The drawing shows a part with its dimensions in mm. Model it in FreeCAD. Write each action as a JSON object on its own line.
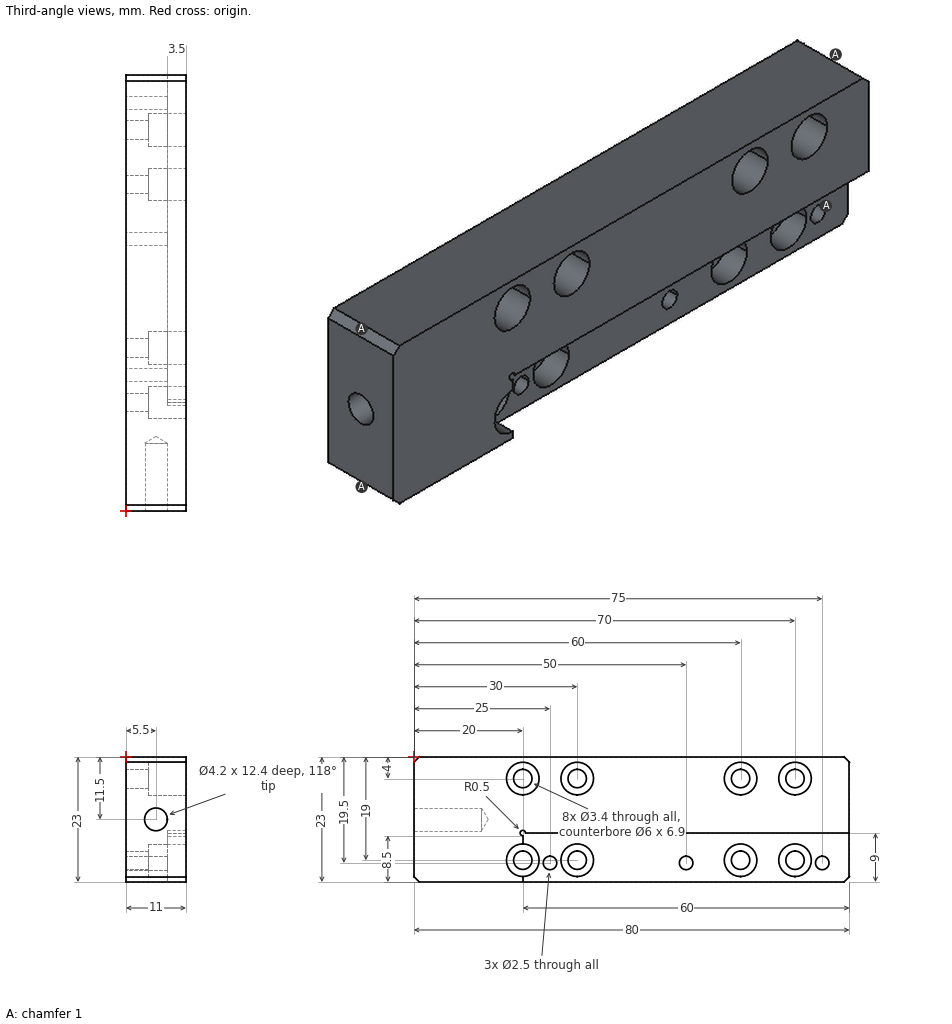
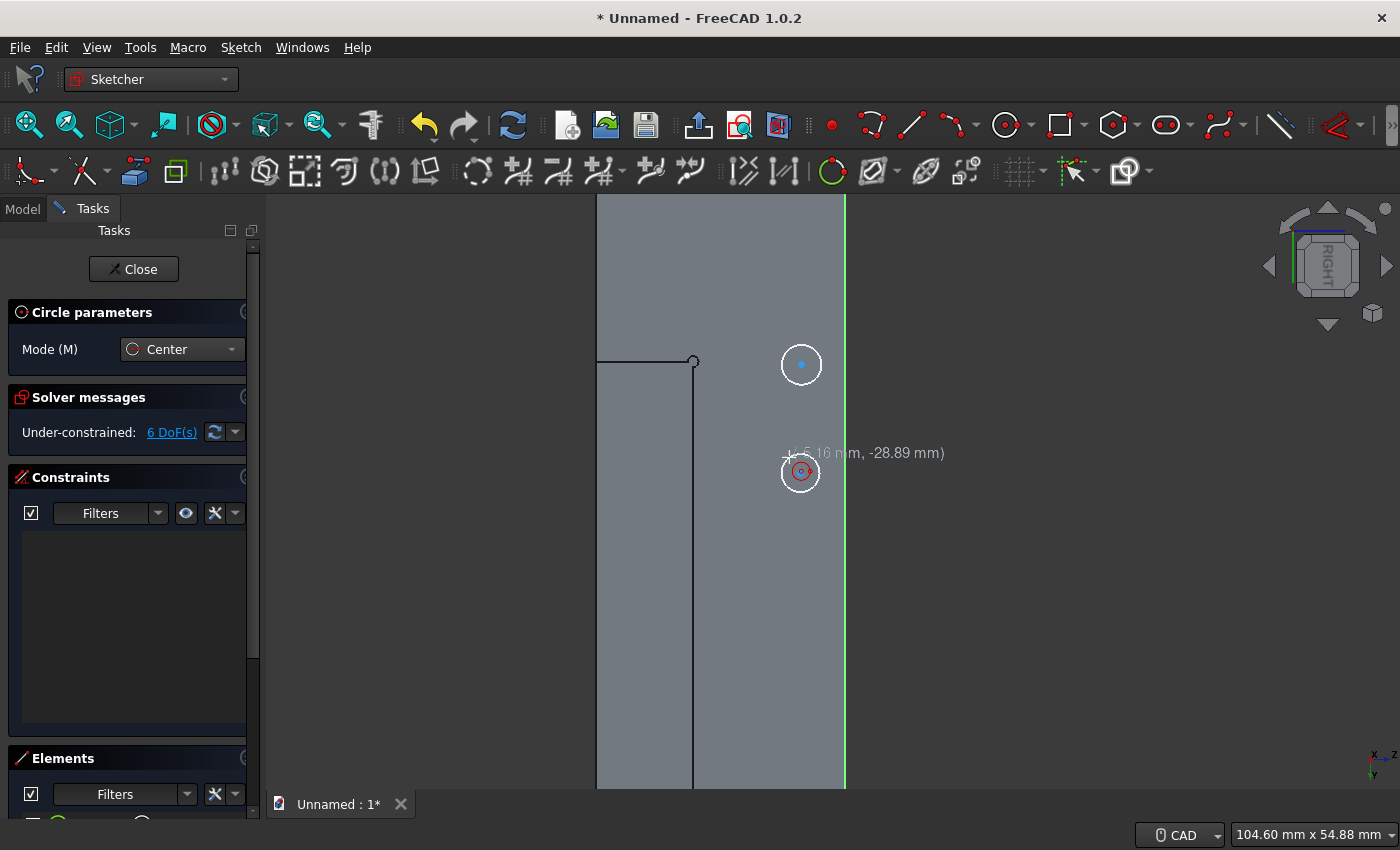
{"action": "scroll", "coordinate": [639, 470], "scroll_direction": "up", "scroll_amount": 2}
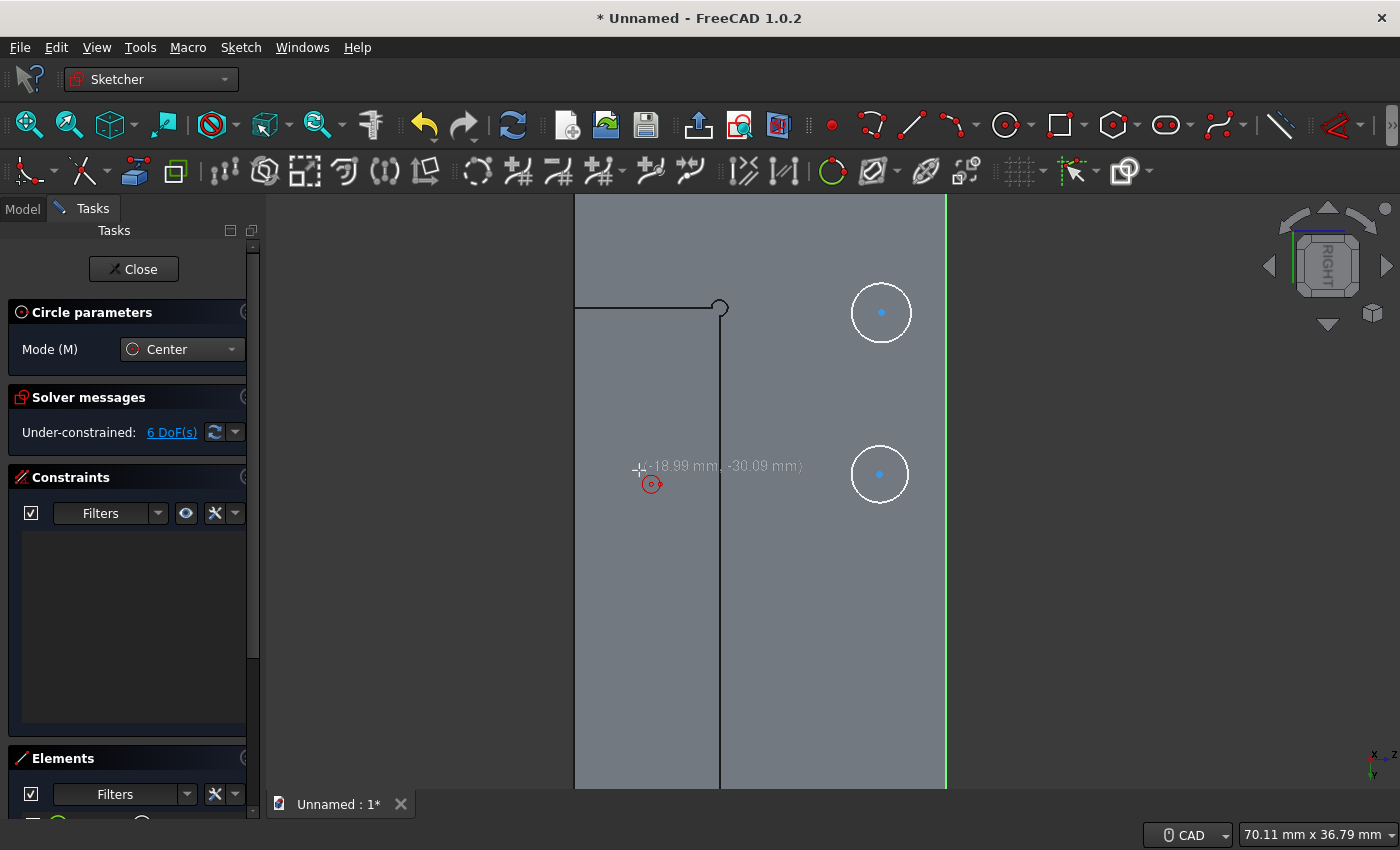
{"action": "scroll", "coordinate": [758, 460], "scroll_direction": "down", "scroll_amount": 6}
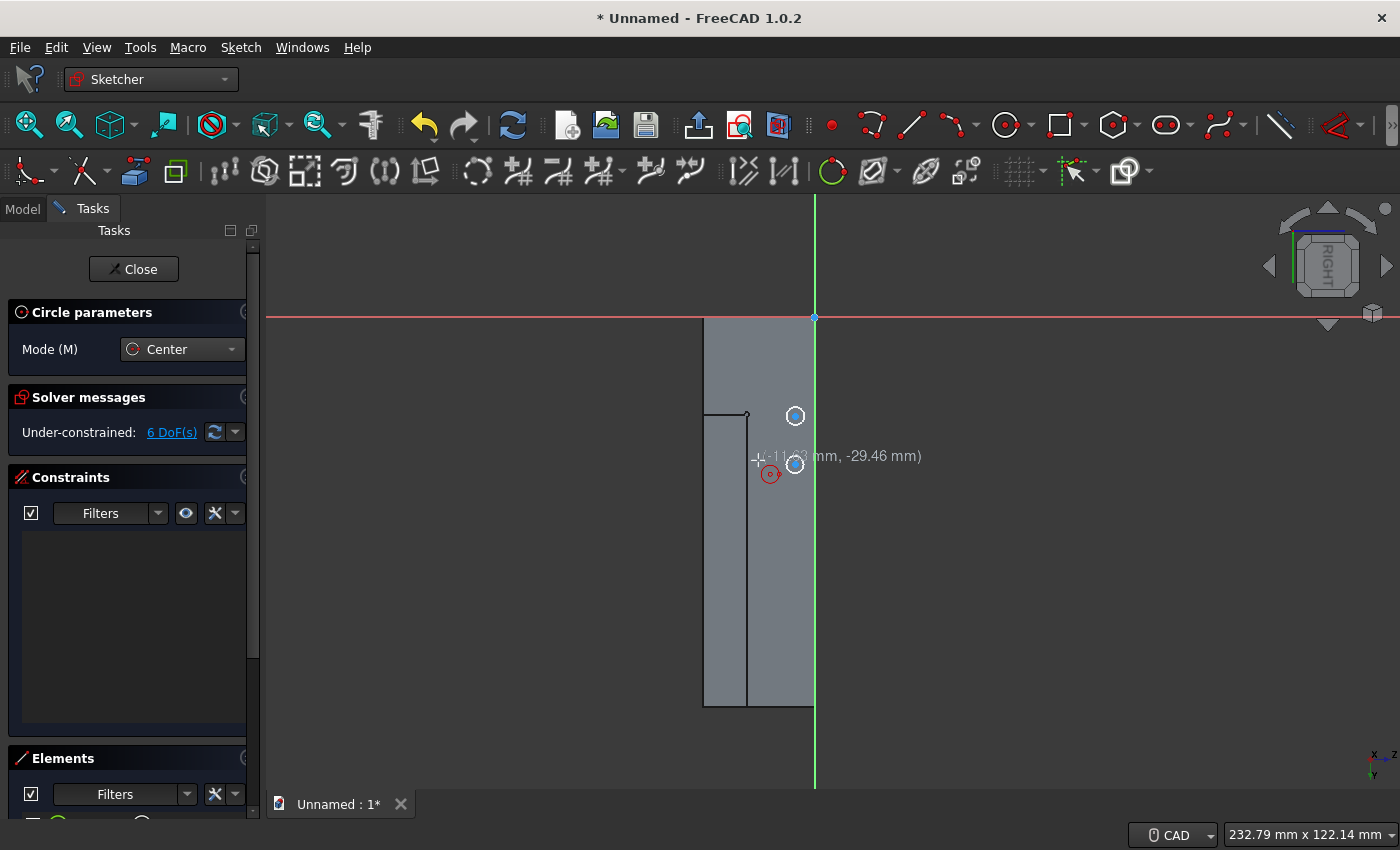
{"action": "left_click", "coordinate": [722, 463]}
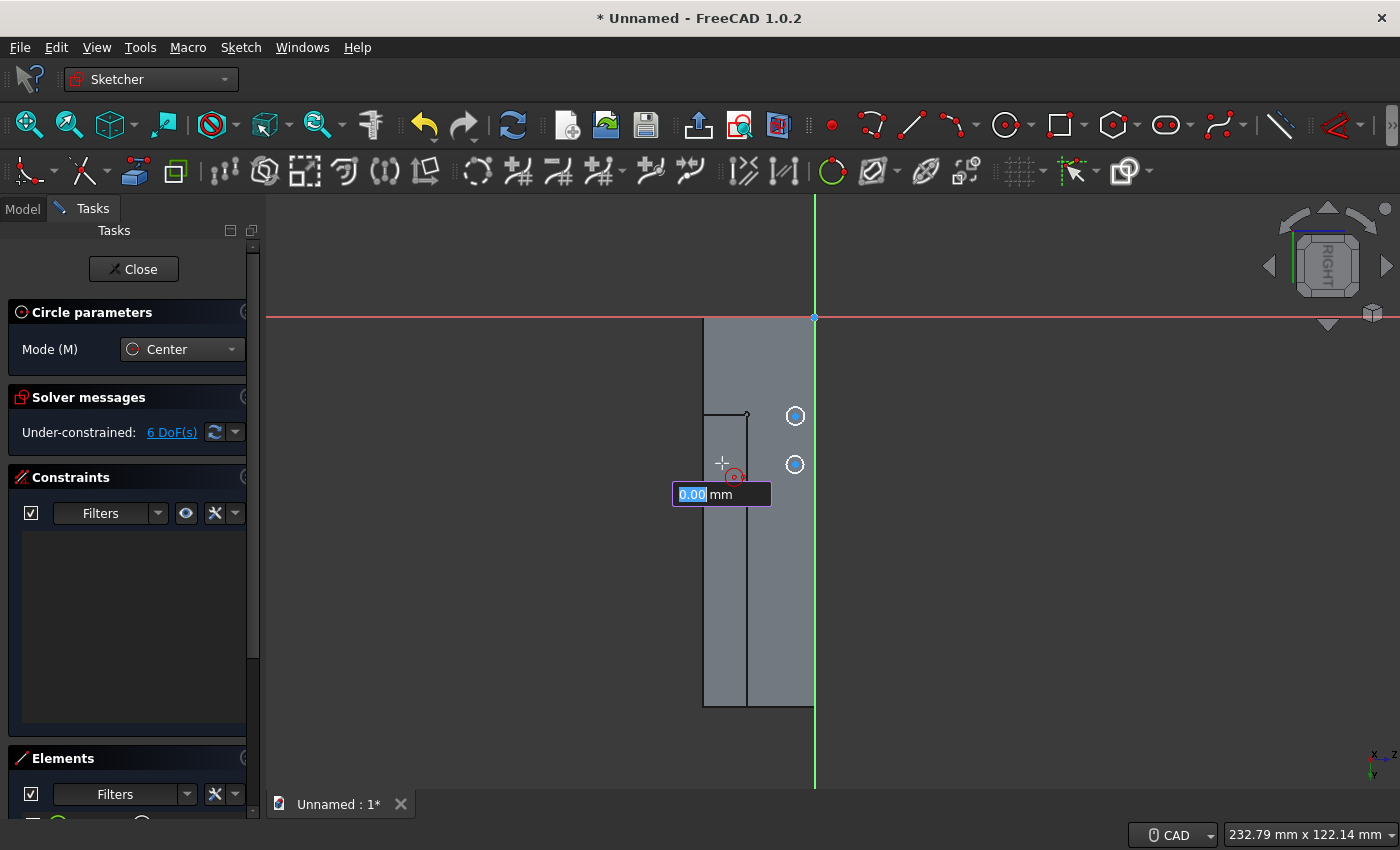
{"action": "scroll", "coordinate": [728, 457], "scroll_direction": "up", "scroll_amount": 4}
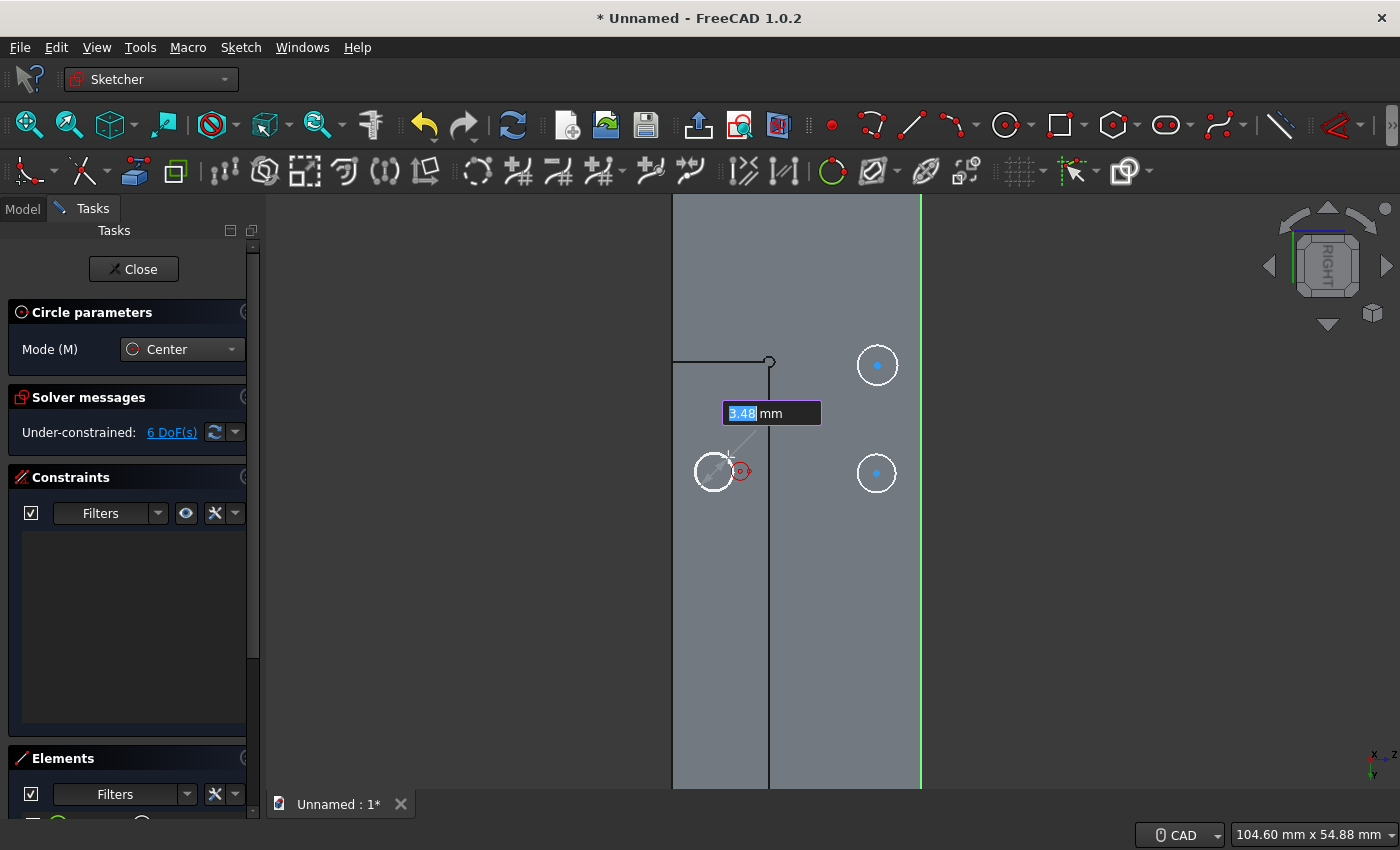
{"action": "left_click", "coordinate": [728, 457]}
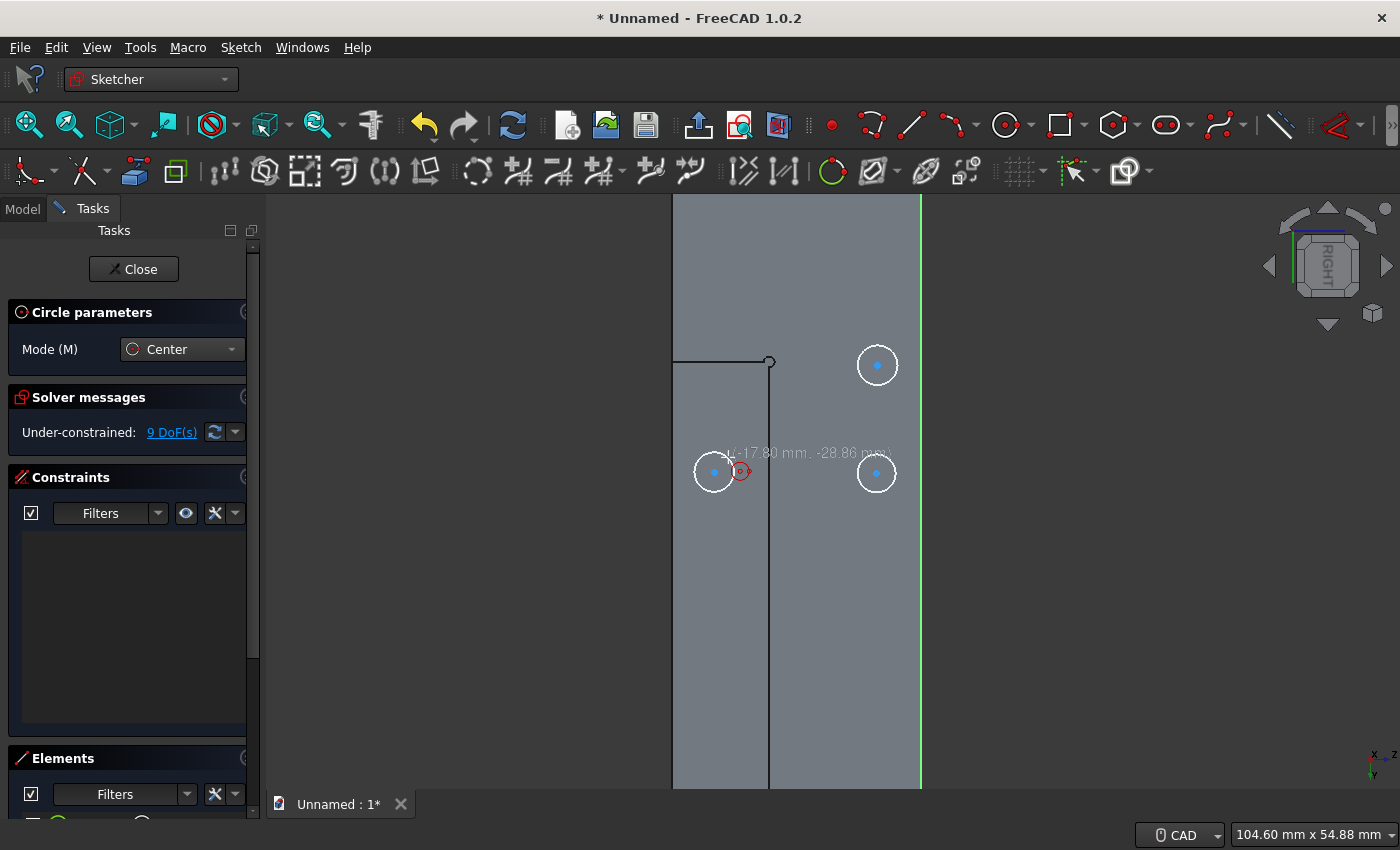
{"action": "scroll", "coordinate": [715, 362], "scroll_direction": "up", "scroll_amount": 2}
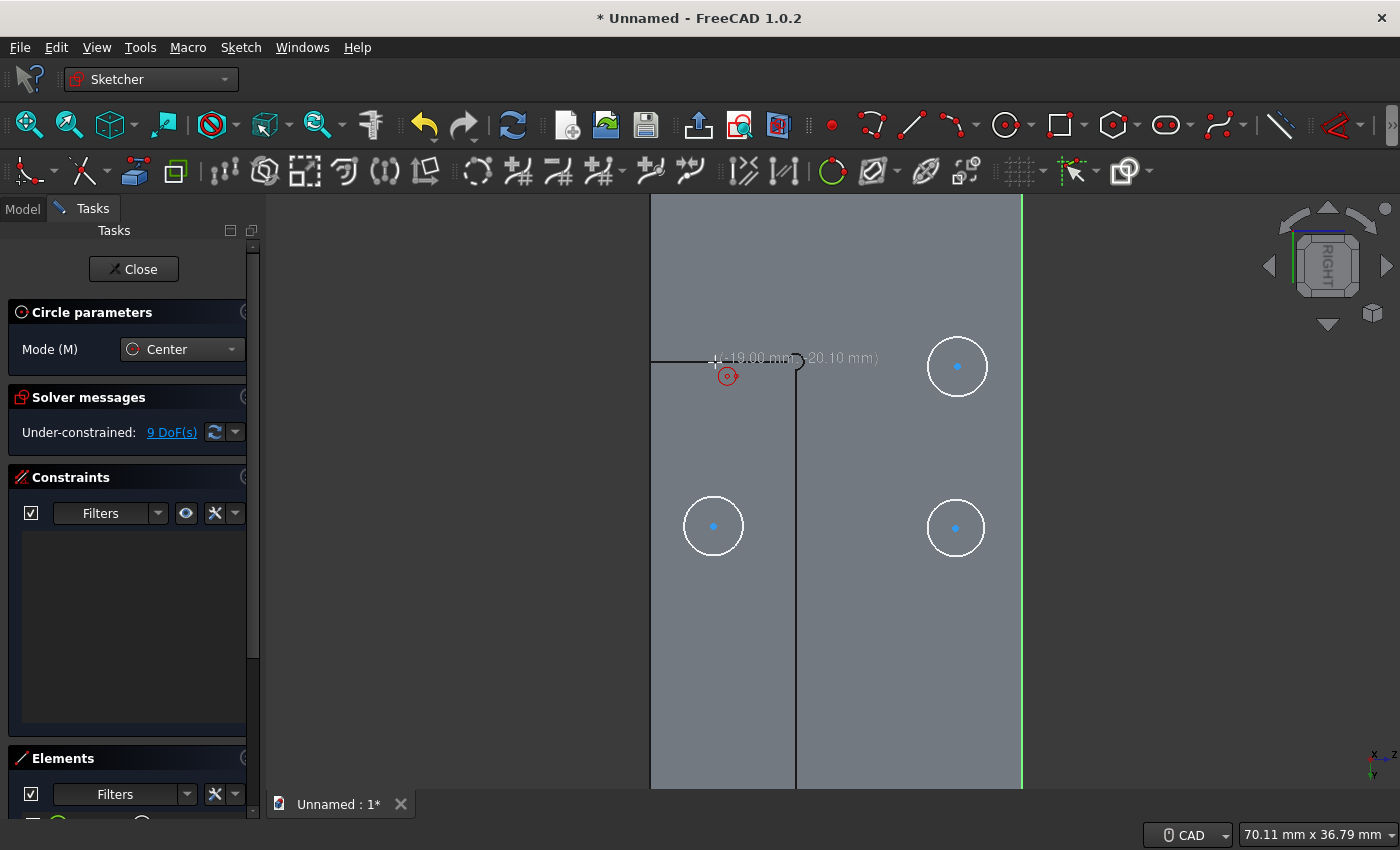
{"action": "scroll", "coordinate": [726, 437], "scroll_direction": "down", "scroll_amount": 6}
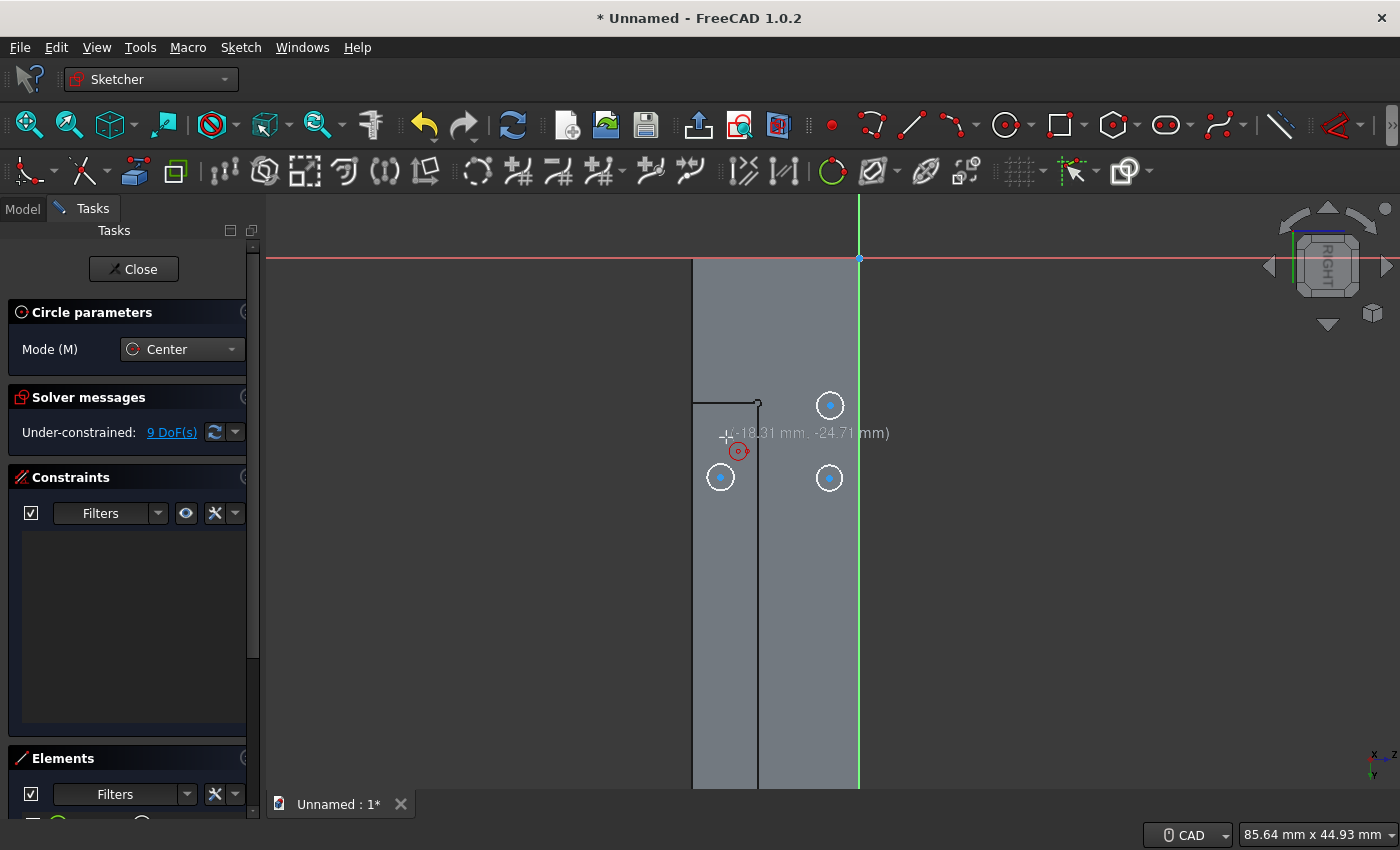
{"action": "left_click", "coordinate": [723, 415]}